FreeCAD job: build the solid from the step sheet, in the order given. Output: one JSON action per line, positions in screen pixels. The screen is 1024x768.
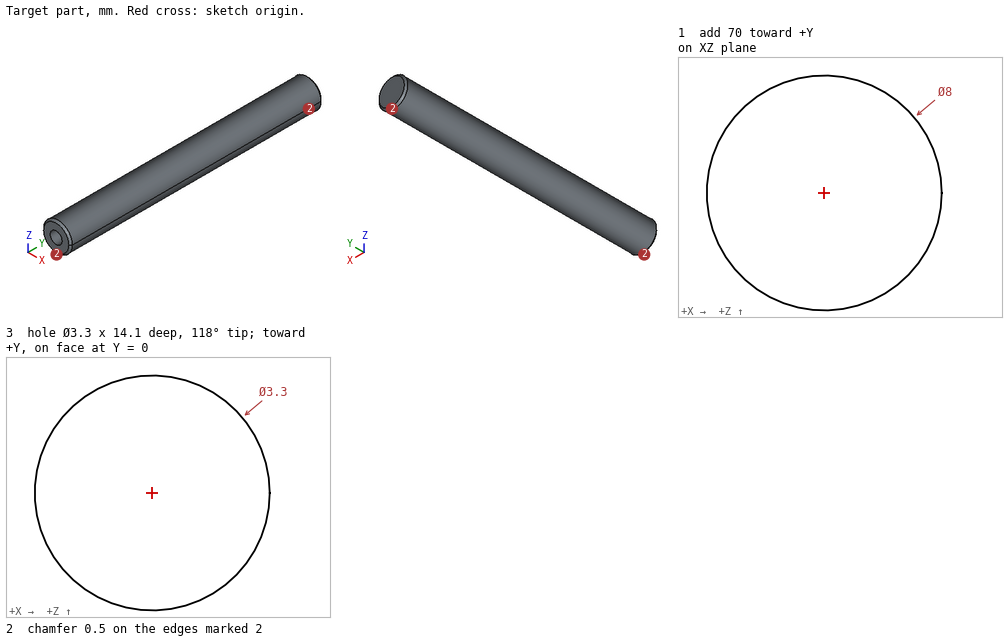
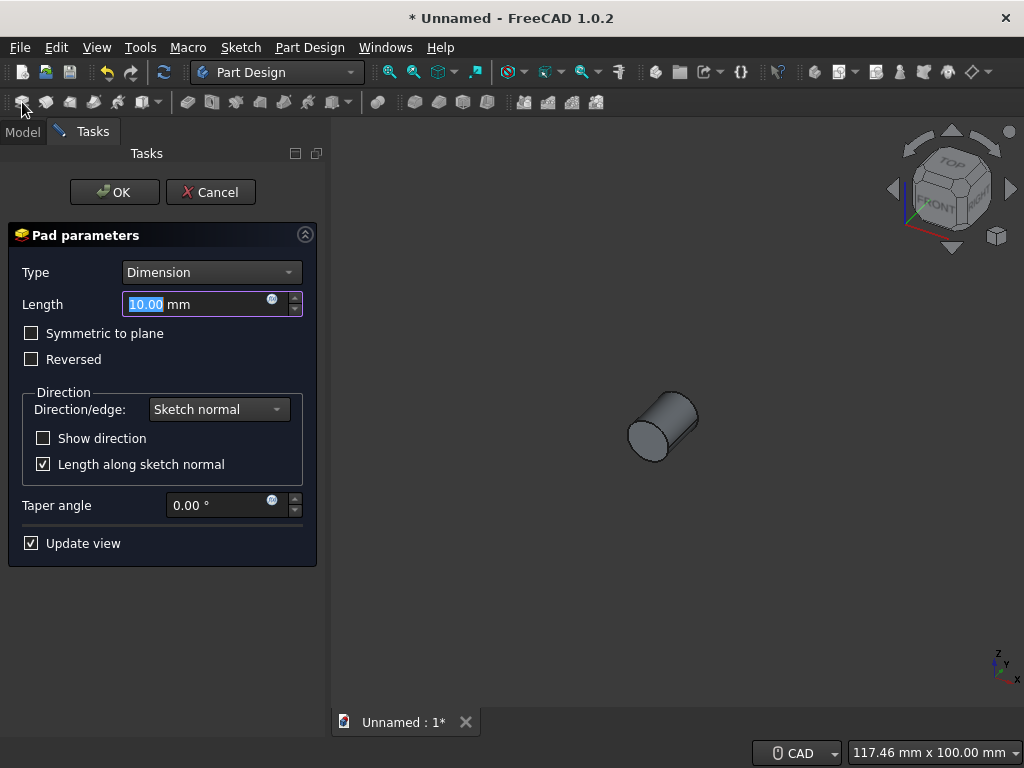
{"action": "type", "text": "70"}
{"action": "key", "text": "Tab"}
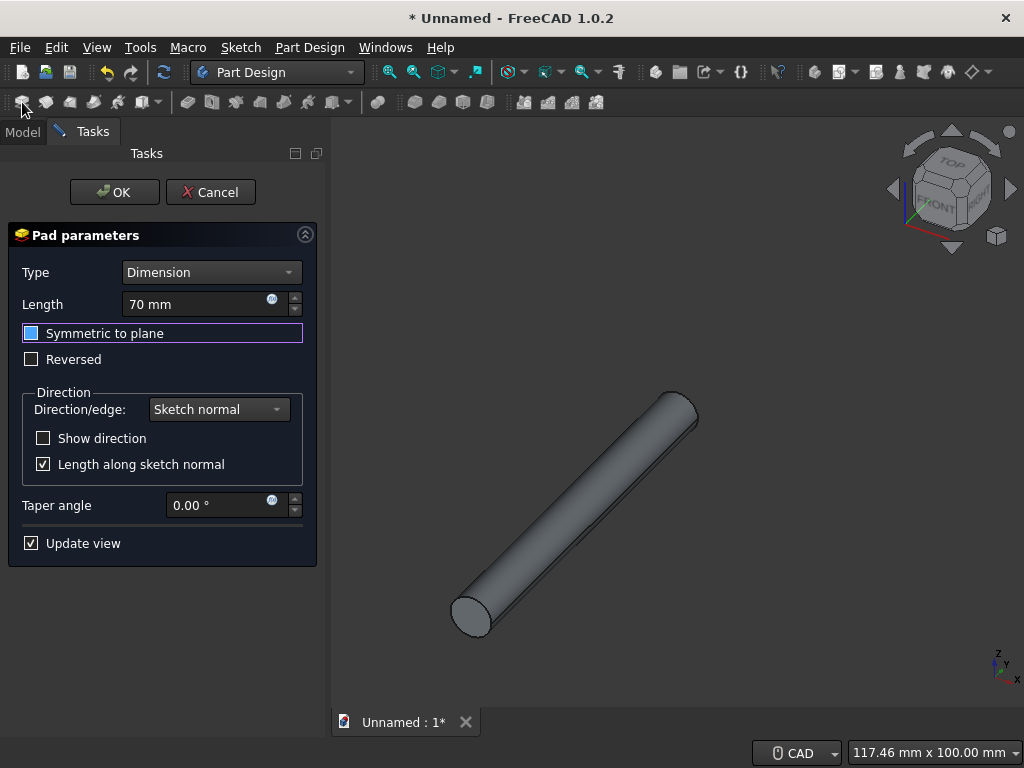
{"action": "left_click", "coordinate": [30, 359]}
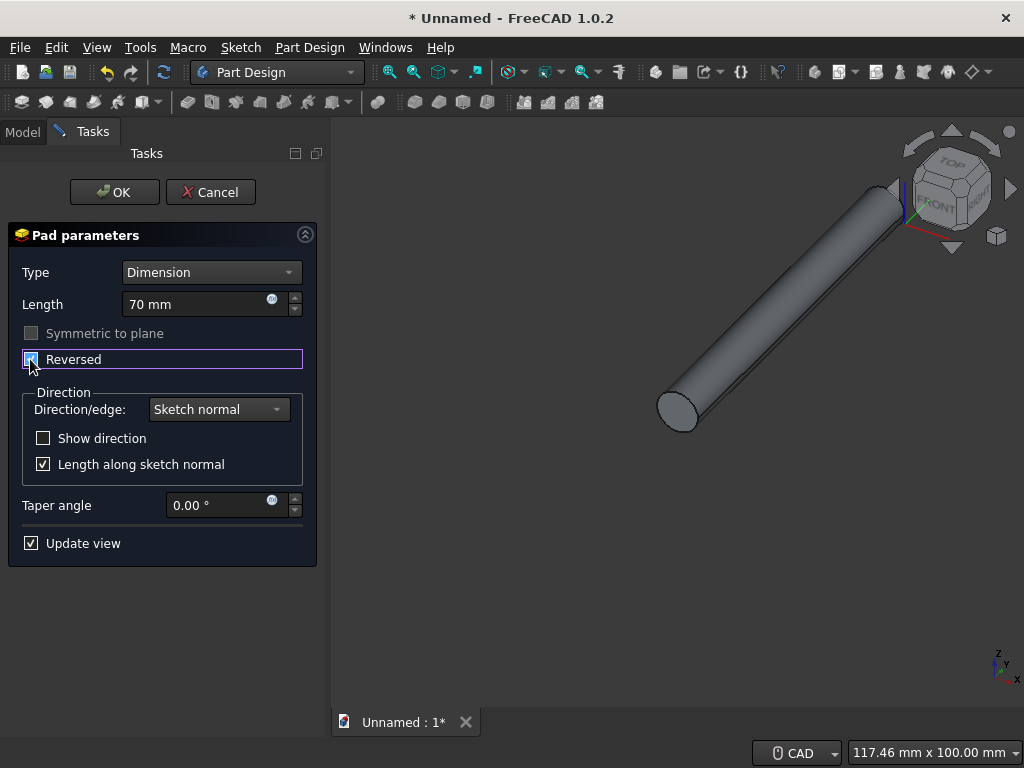
{"action": "left_click", "coordinate": [115, 192]}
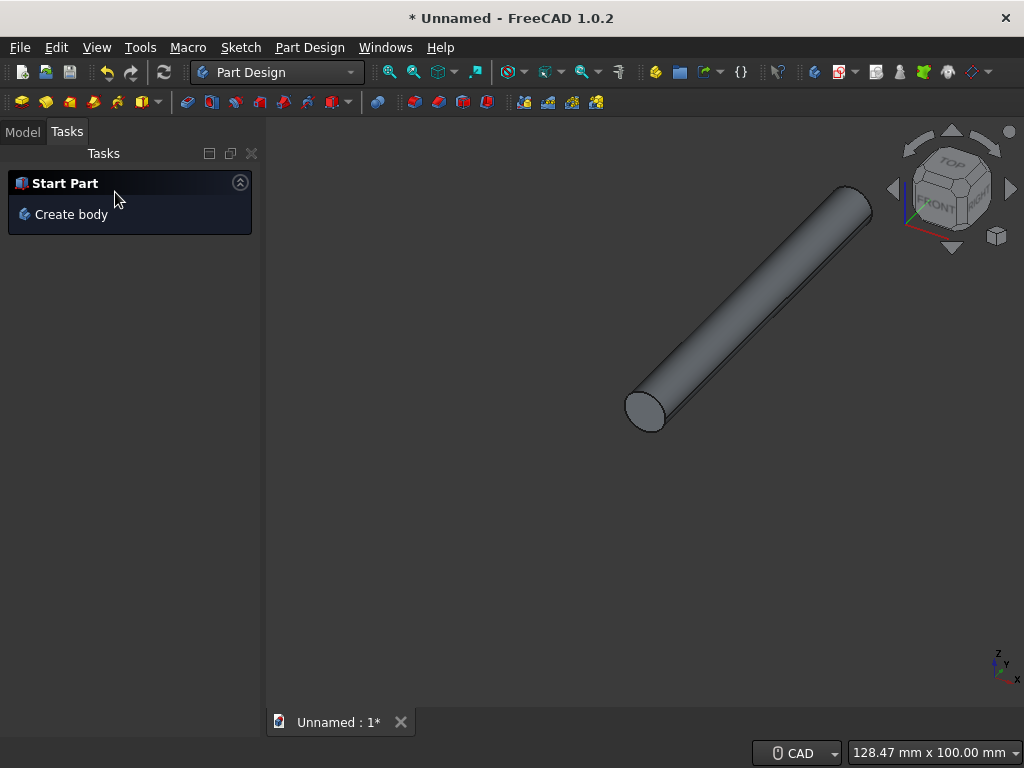
{"action": "left_click", "coordinate": [390, 72]}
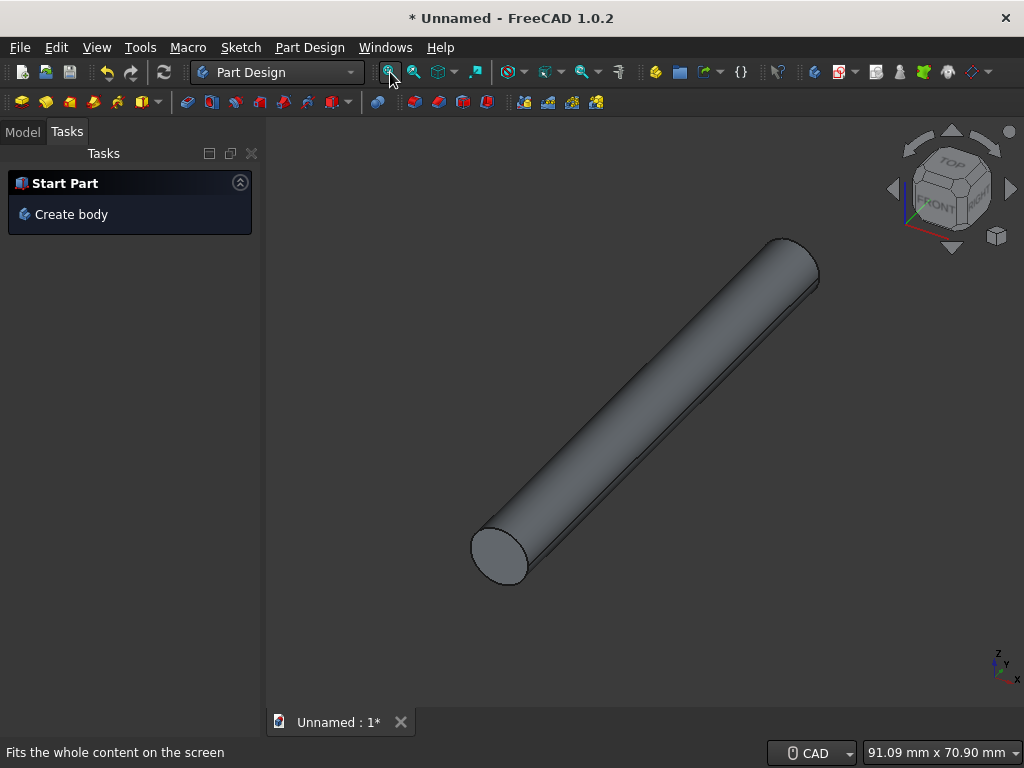
{"action": "left_click", "coordinate": [476, 532]}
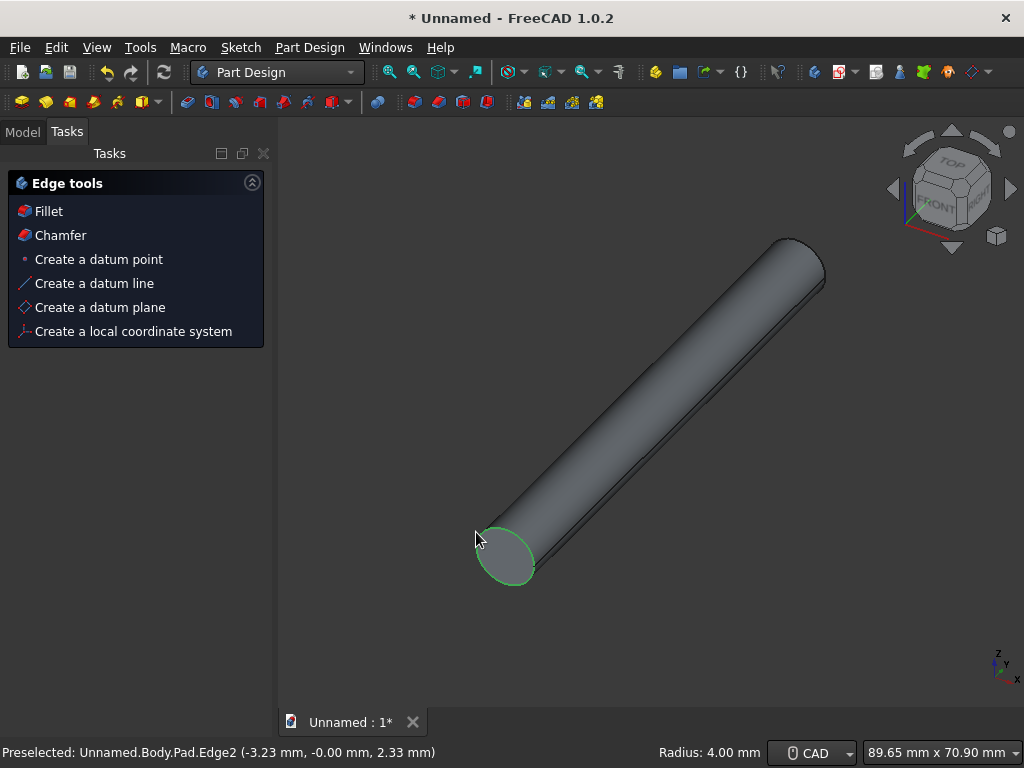
{"action": "key", "text": "0"}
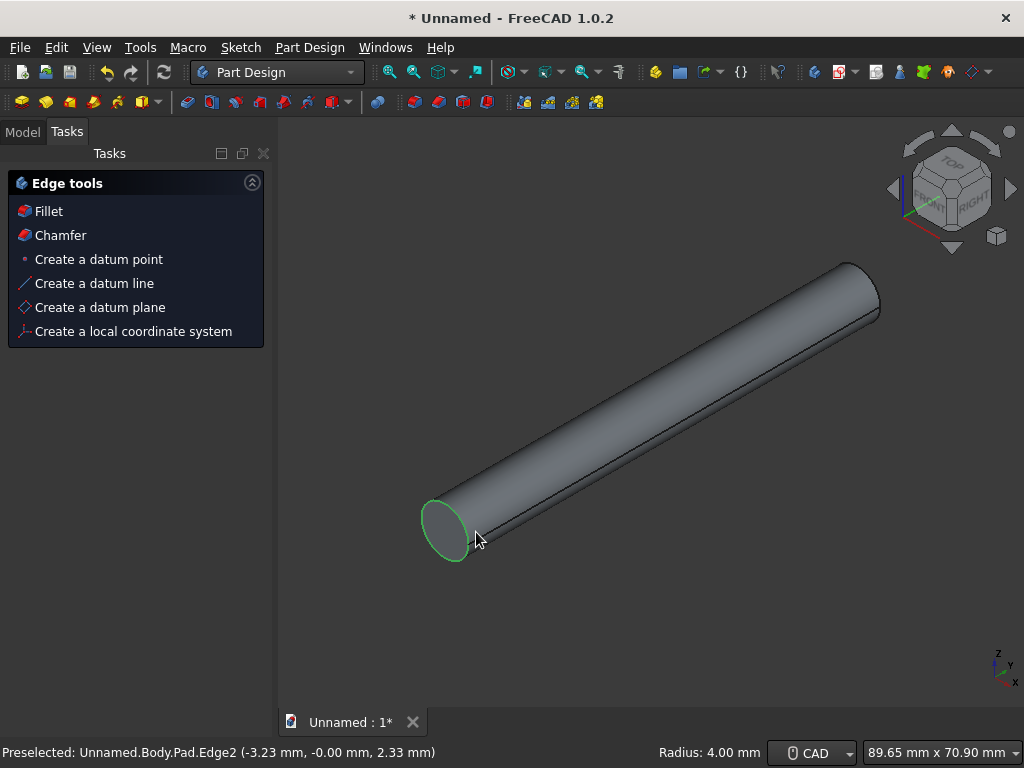
{"action": "key", "text": "2"}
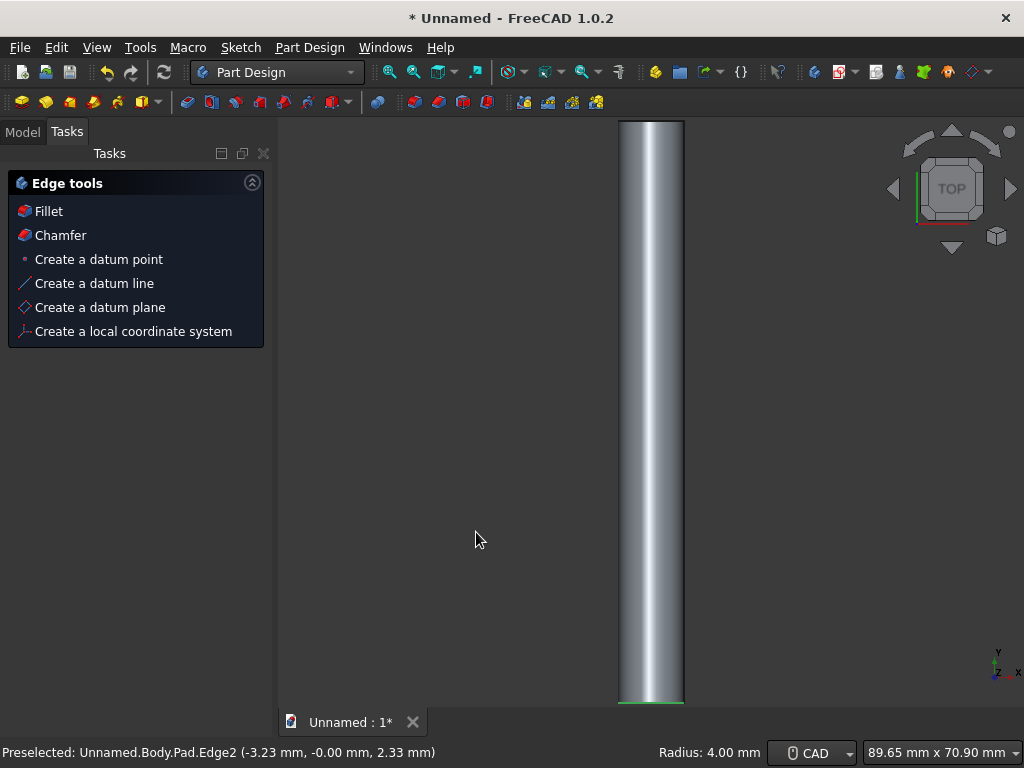
{"action": "key", "text": "1"}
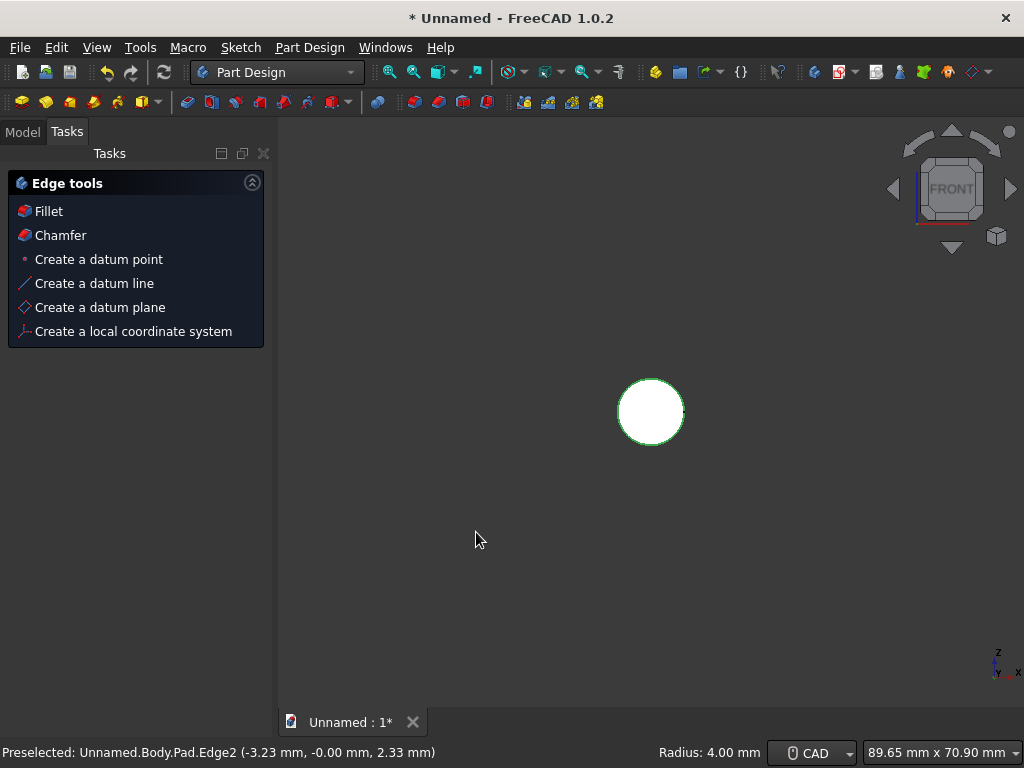
{"action": "left_click", "coordinate": [390, 72]}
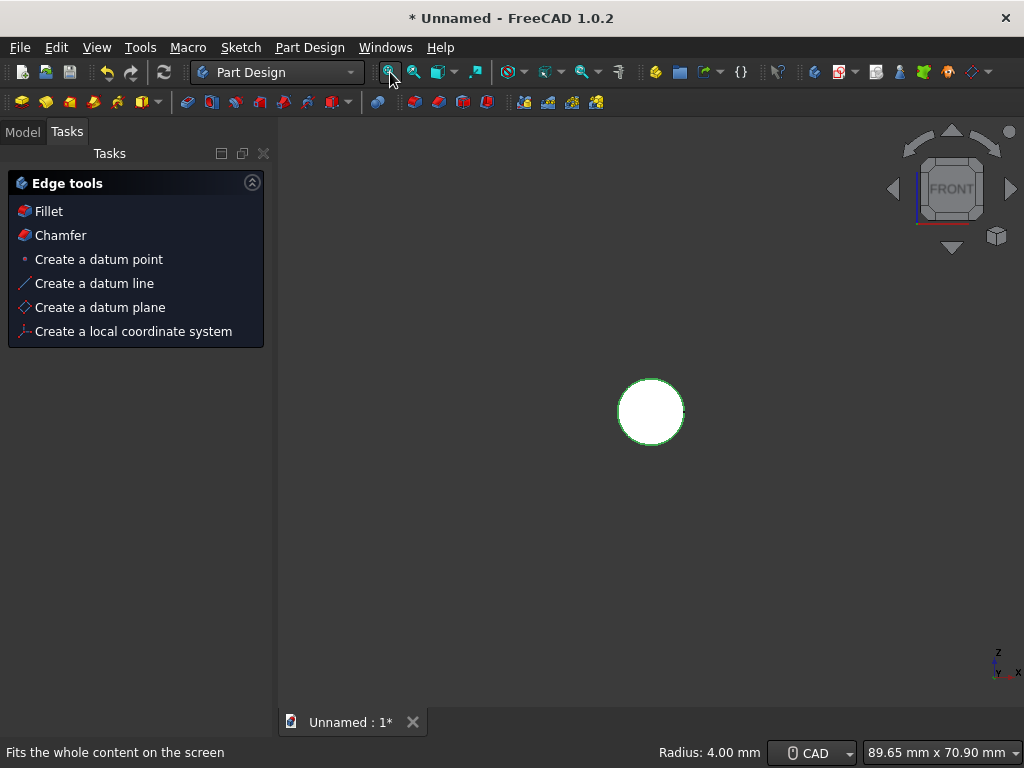
{"action": "key", "text": "3"}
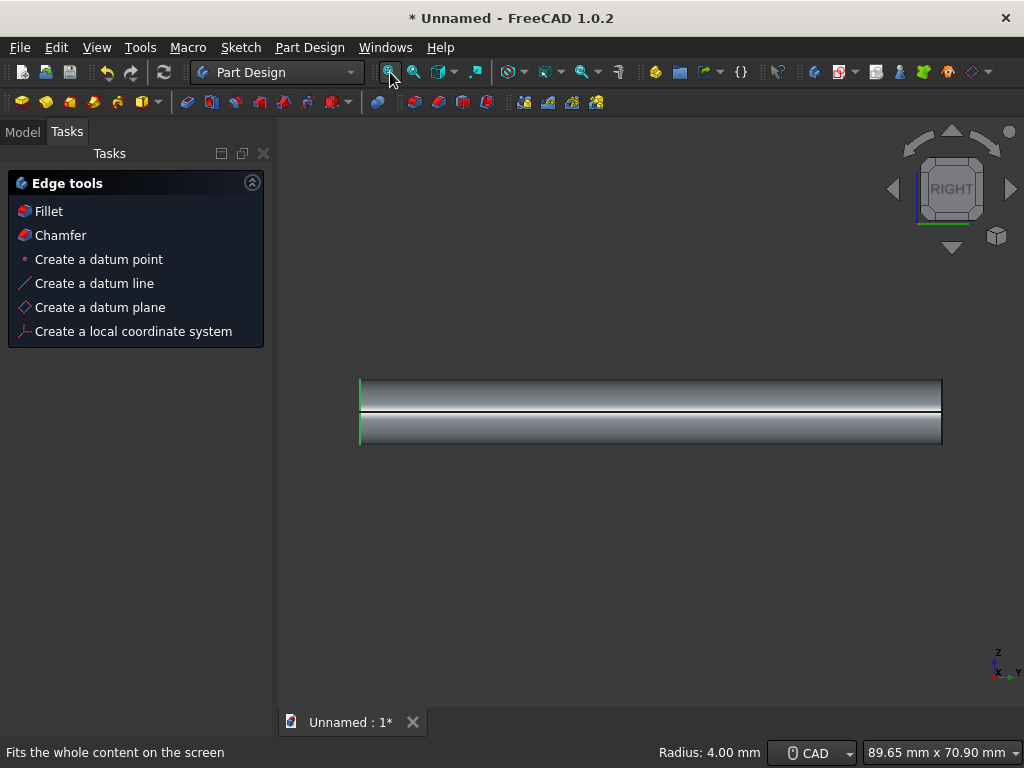
{"action": "left_click", "coordinate": [942, 391], "text": "ctrl"}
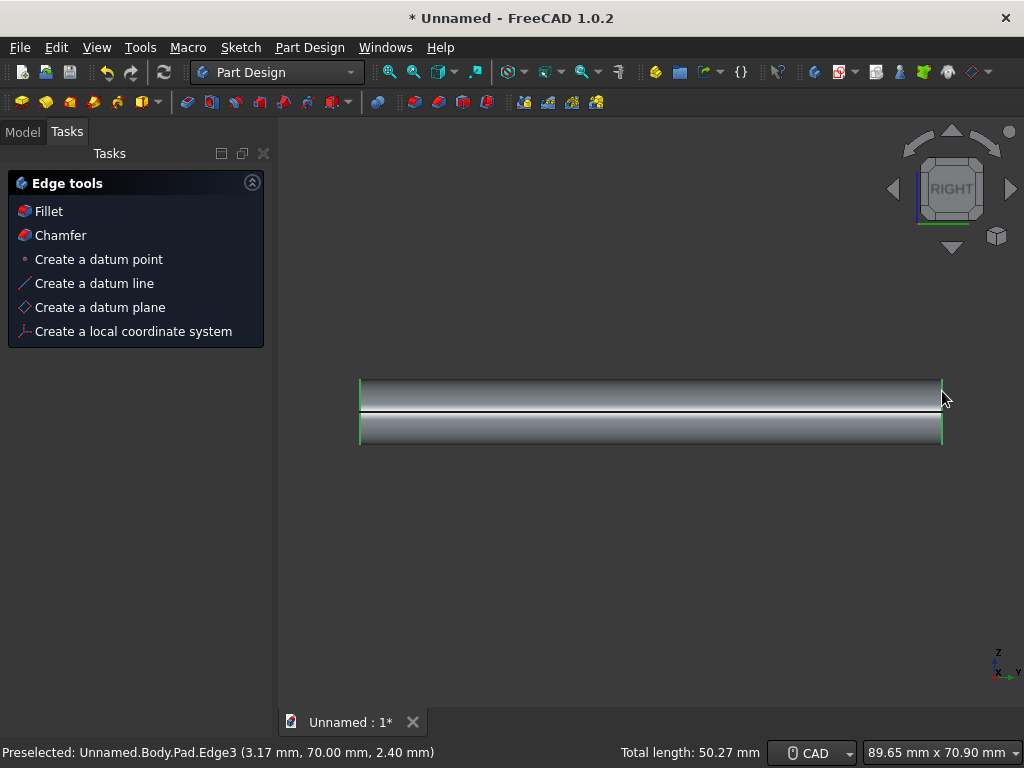
{"action": "left_click", "coordinate": [440, 102]}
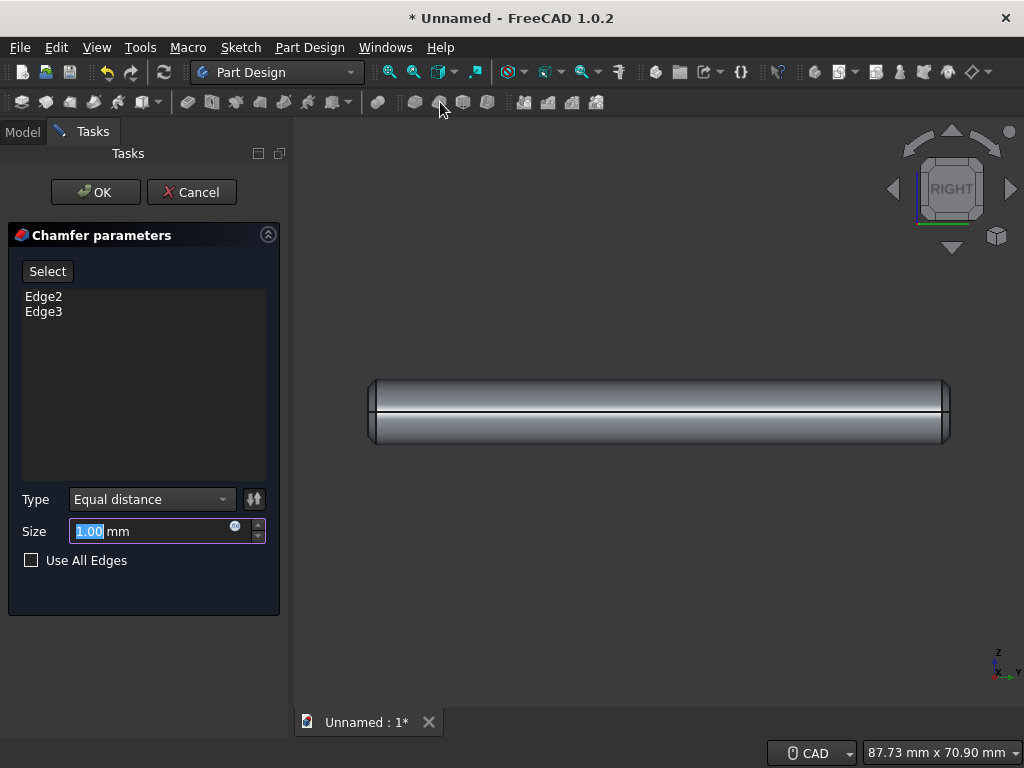
{"action": "type", "text": "0.5"}
{"action": "key", "text": "Tab"}